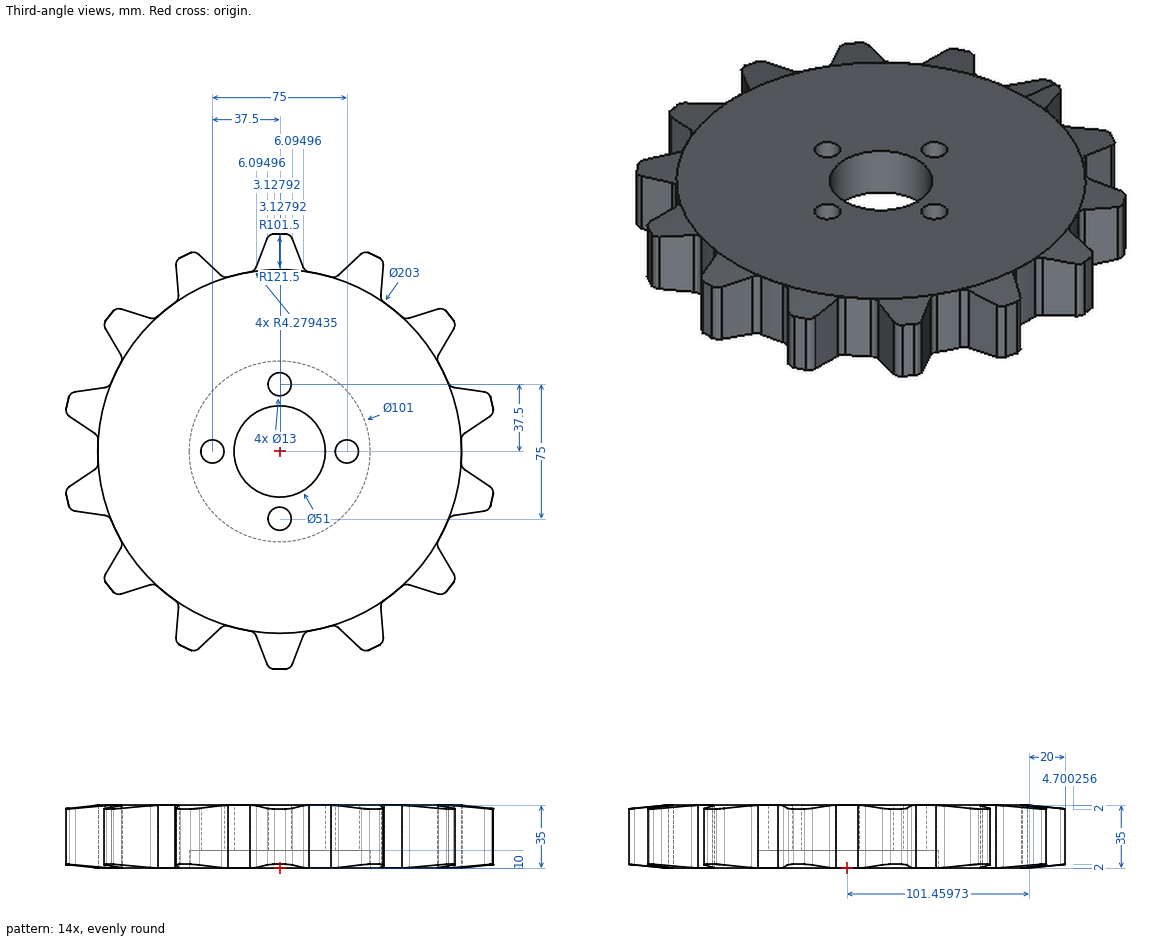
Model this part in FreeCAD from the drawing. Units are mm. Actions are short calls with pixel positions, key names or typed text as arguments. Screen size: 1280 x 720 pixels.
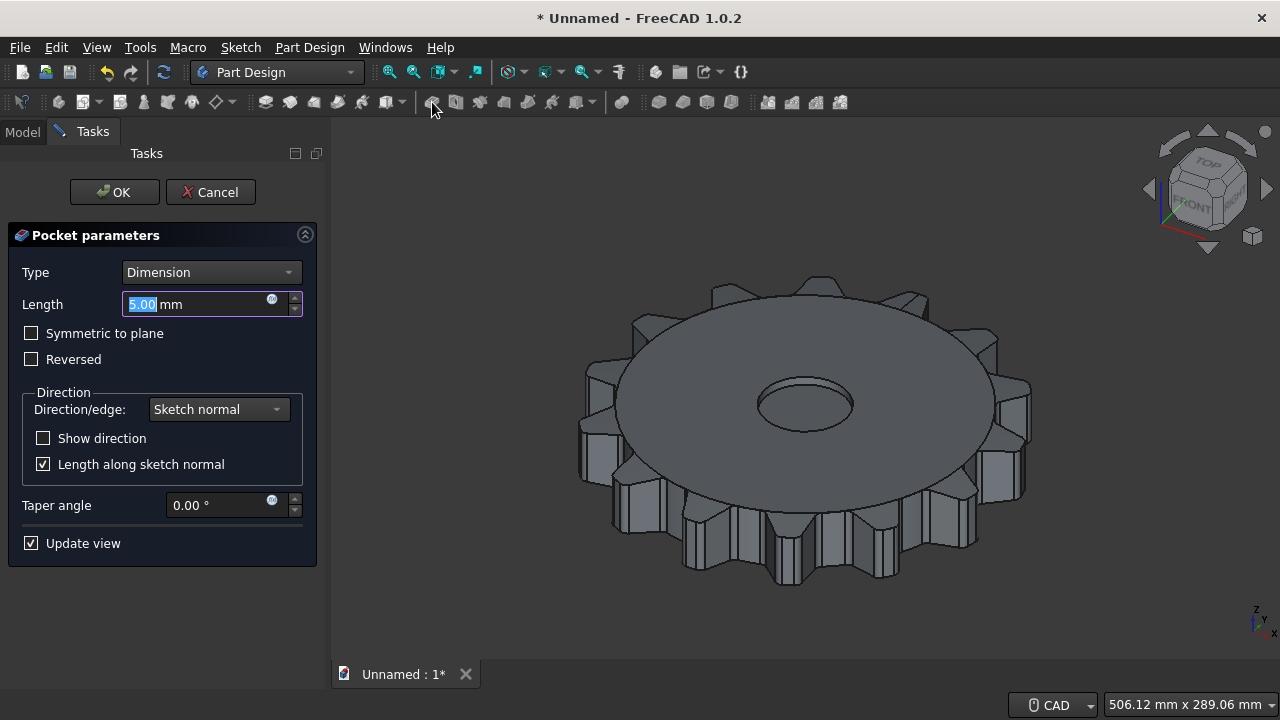
click(212, 272)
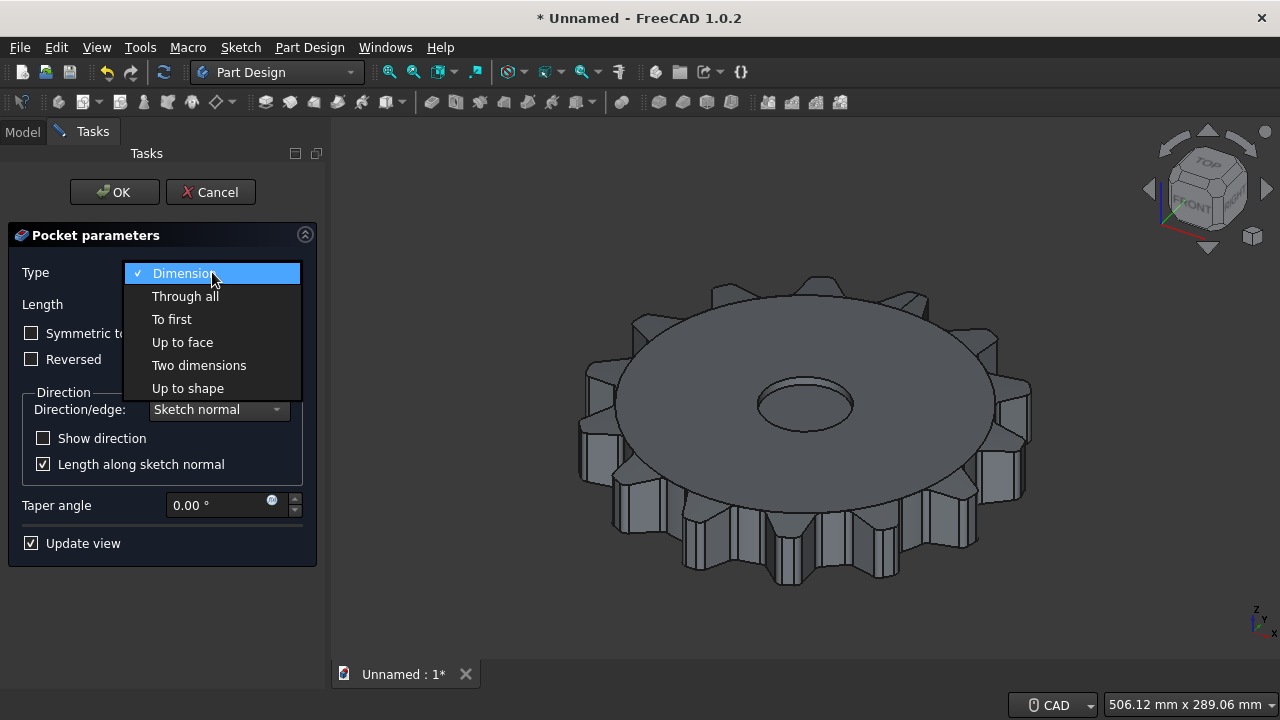
click(212, 296)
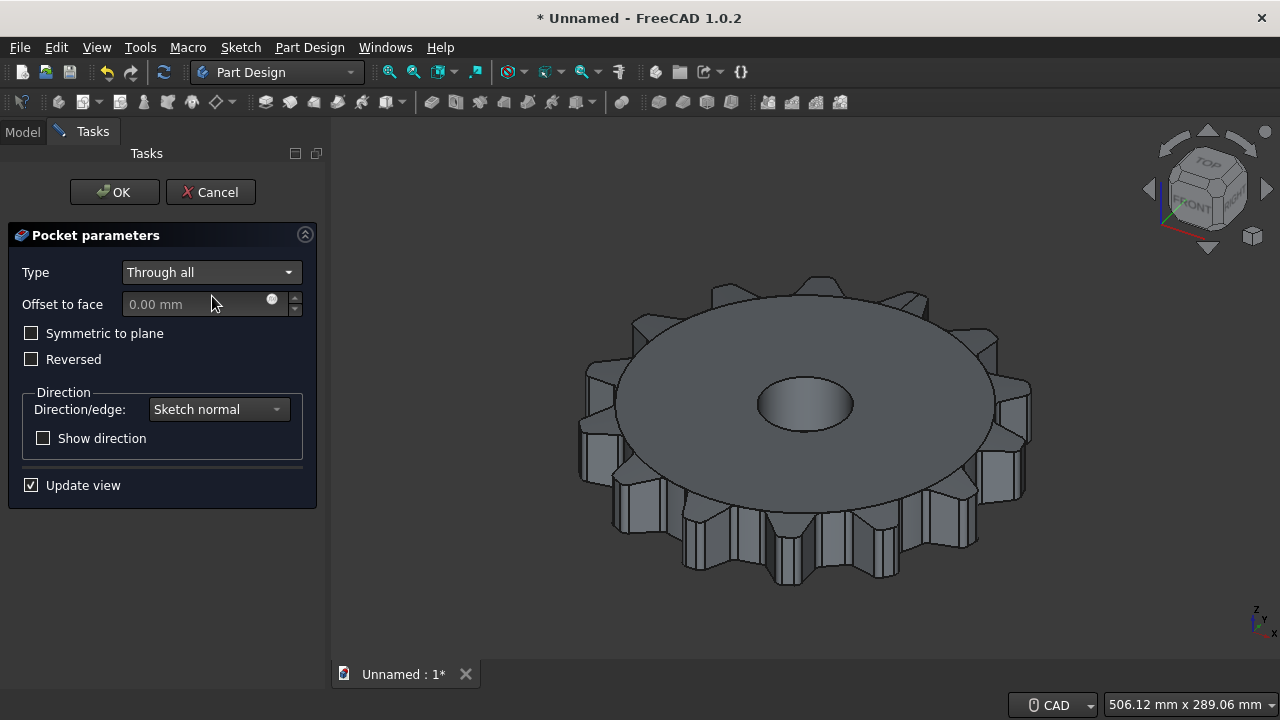
click(115, 192)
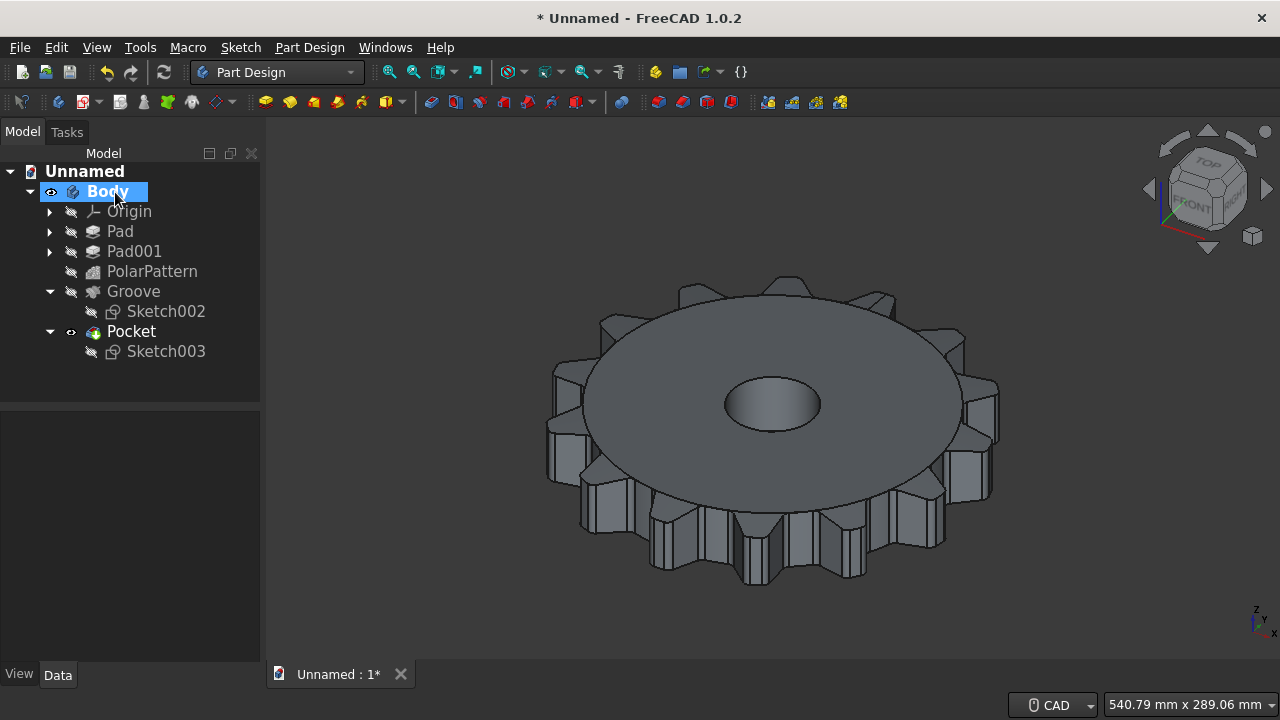
key(5)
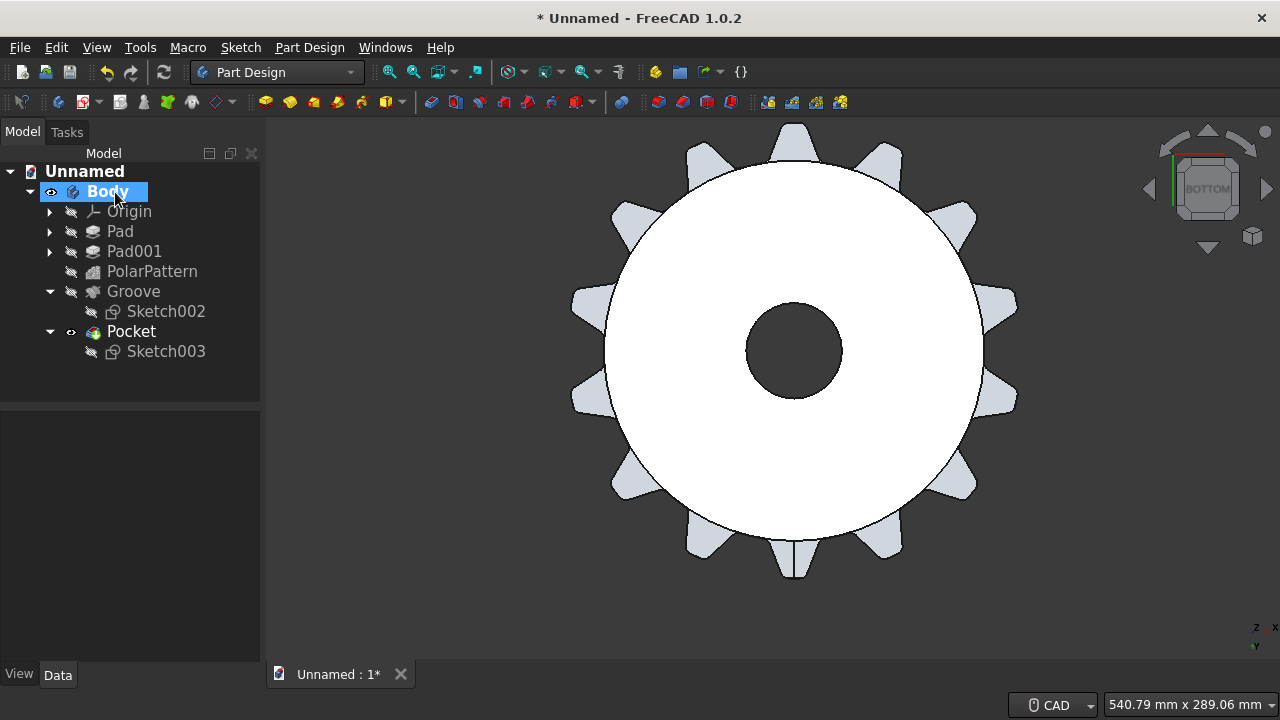
click(903, 404)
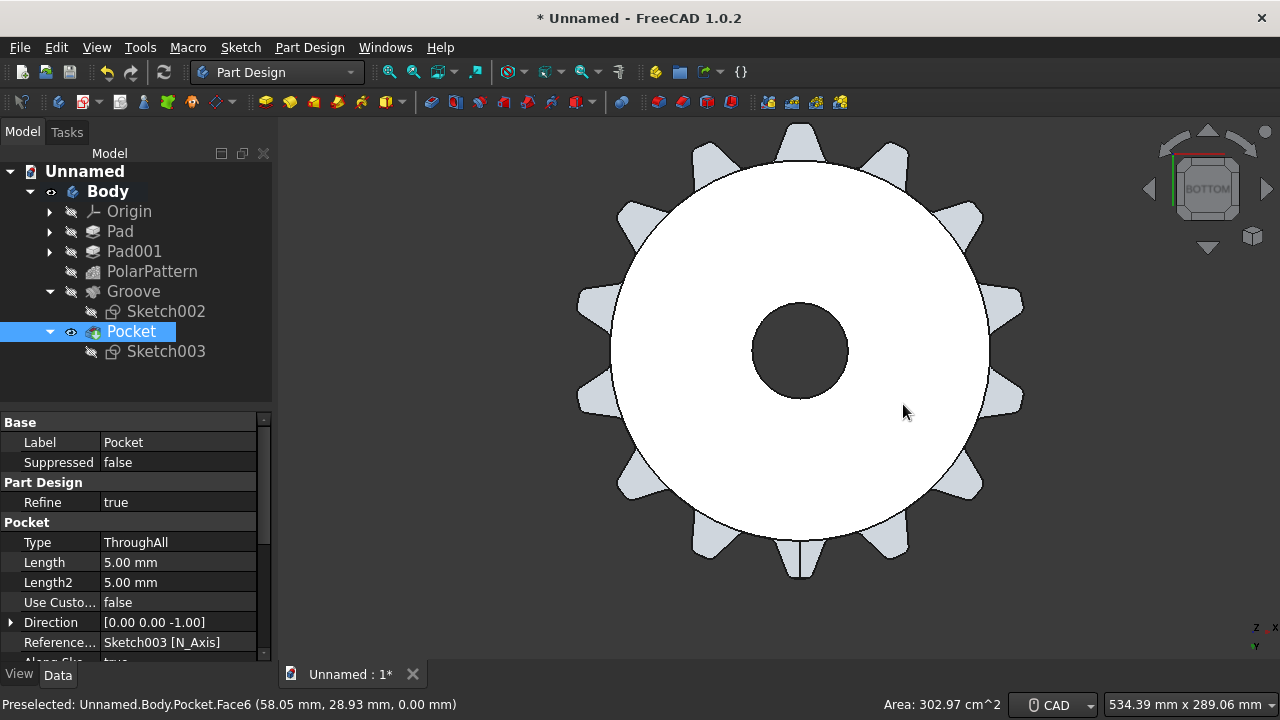
click(84, 102)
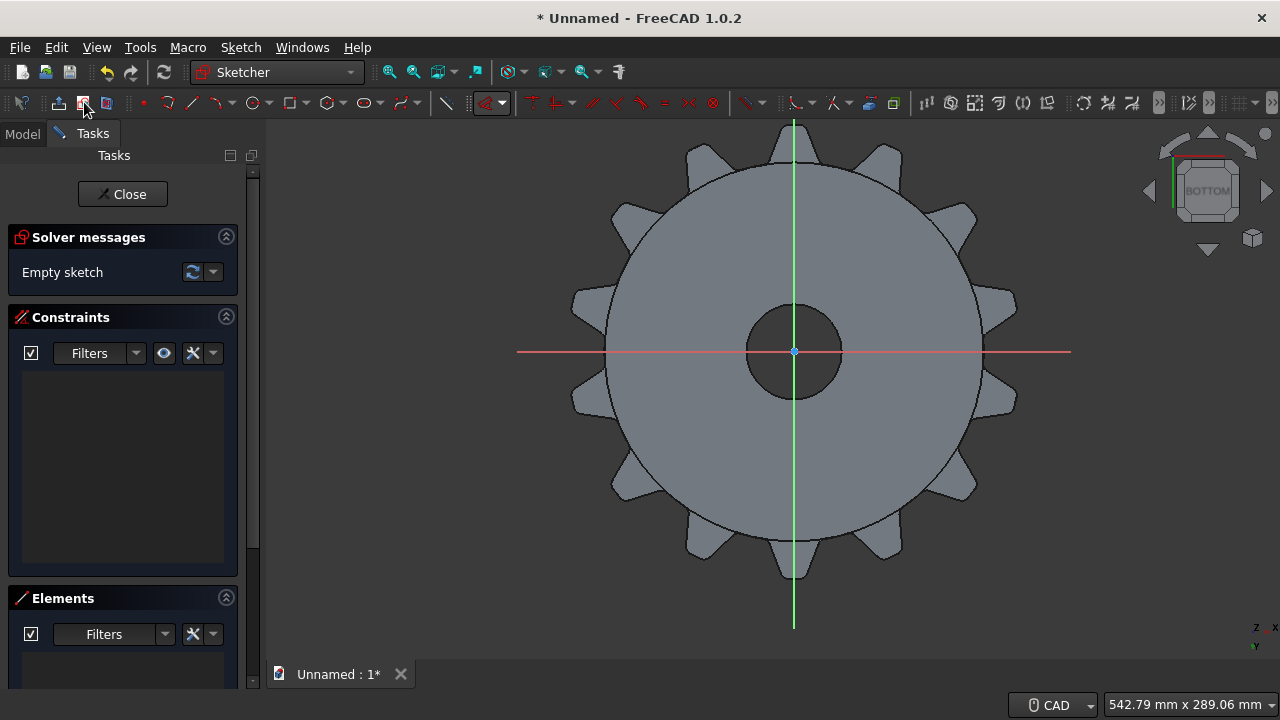
scroll(867, 322, up, 4)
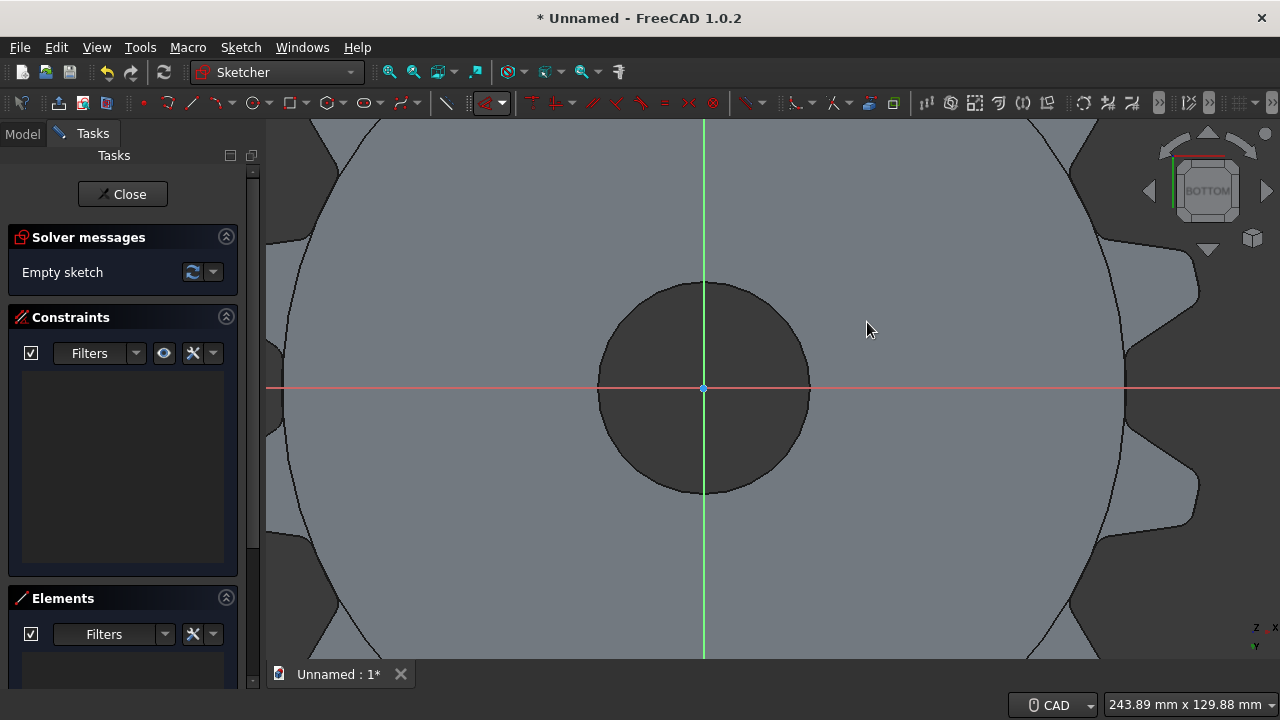
click(254, 104)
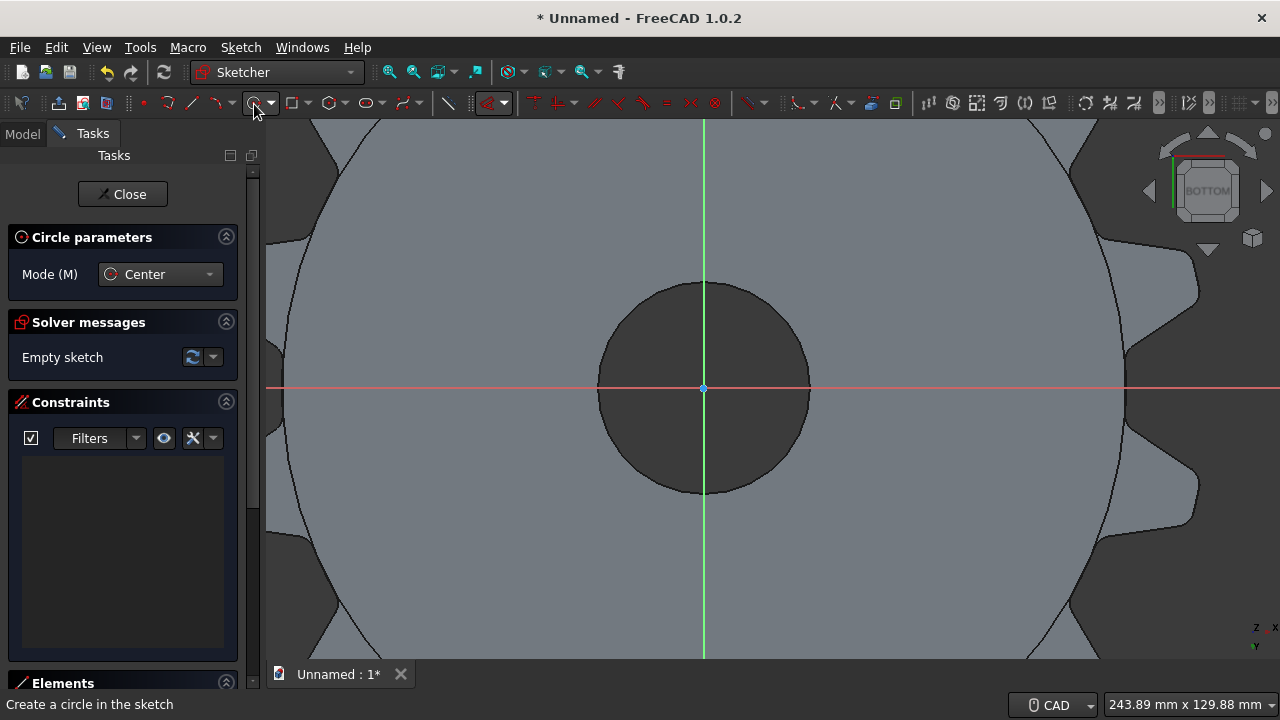
click(704, 544)
move(723, 525)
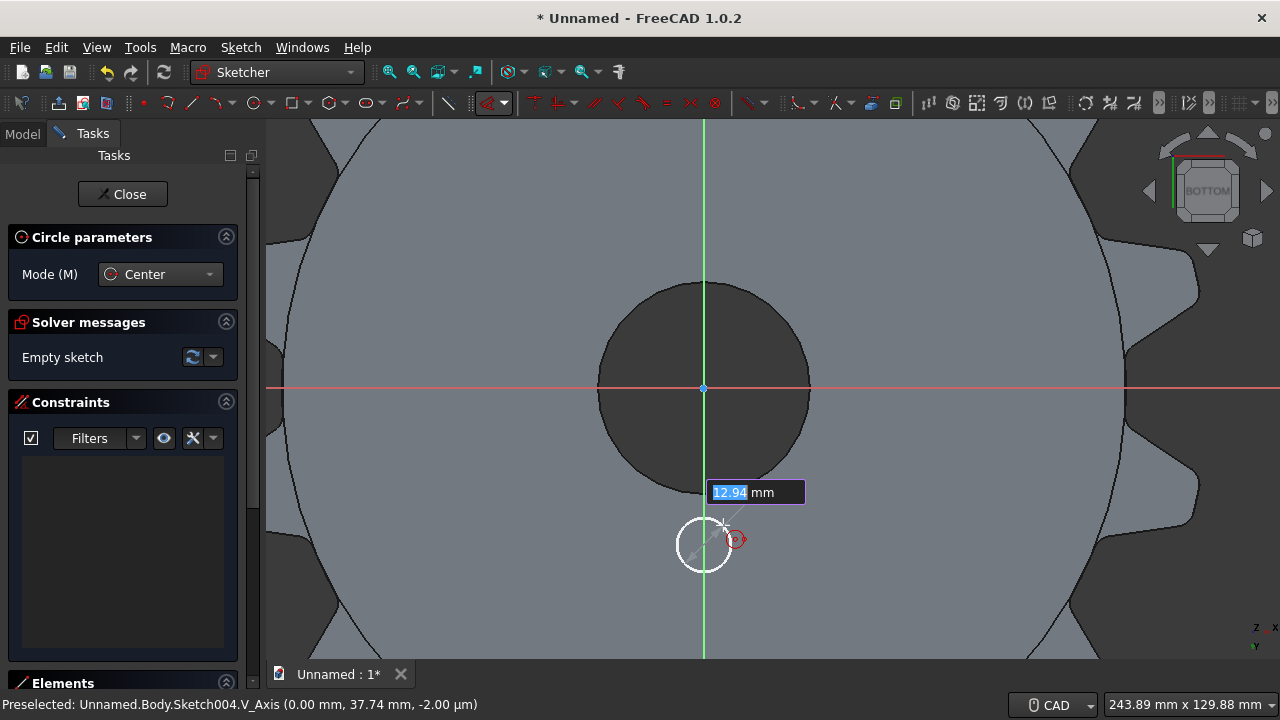
text(13)
key(Return)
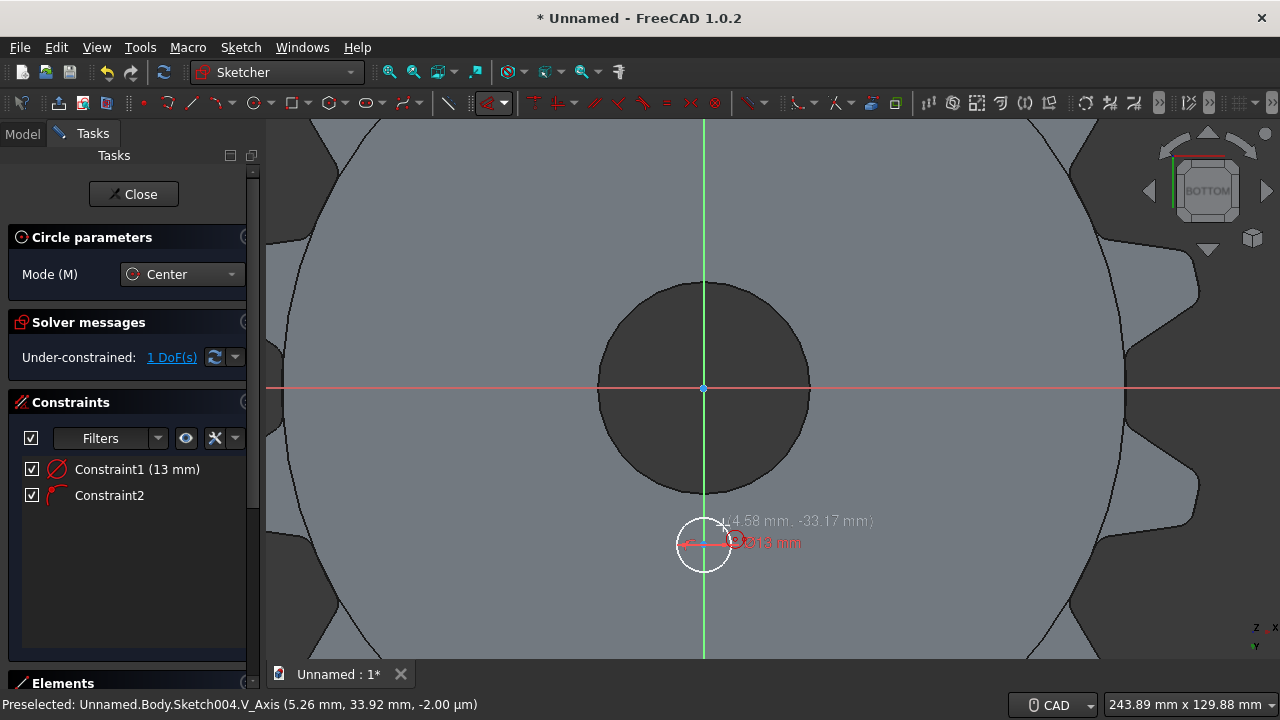
click(548, 388)
move(567, 369)